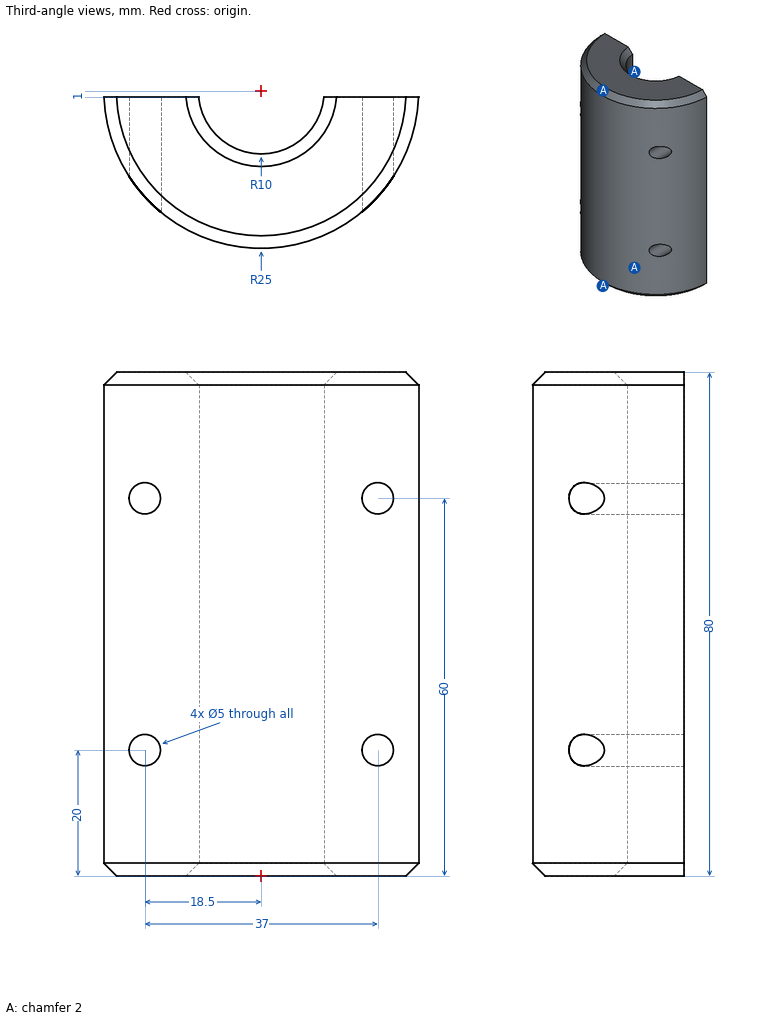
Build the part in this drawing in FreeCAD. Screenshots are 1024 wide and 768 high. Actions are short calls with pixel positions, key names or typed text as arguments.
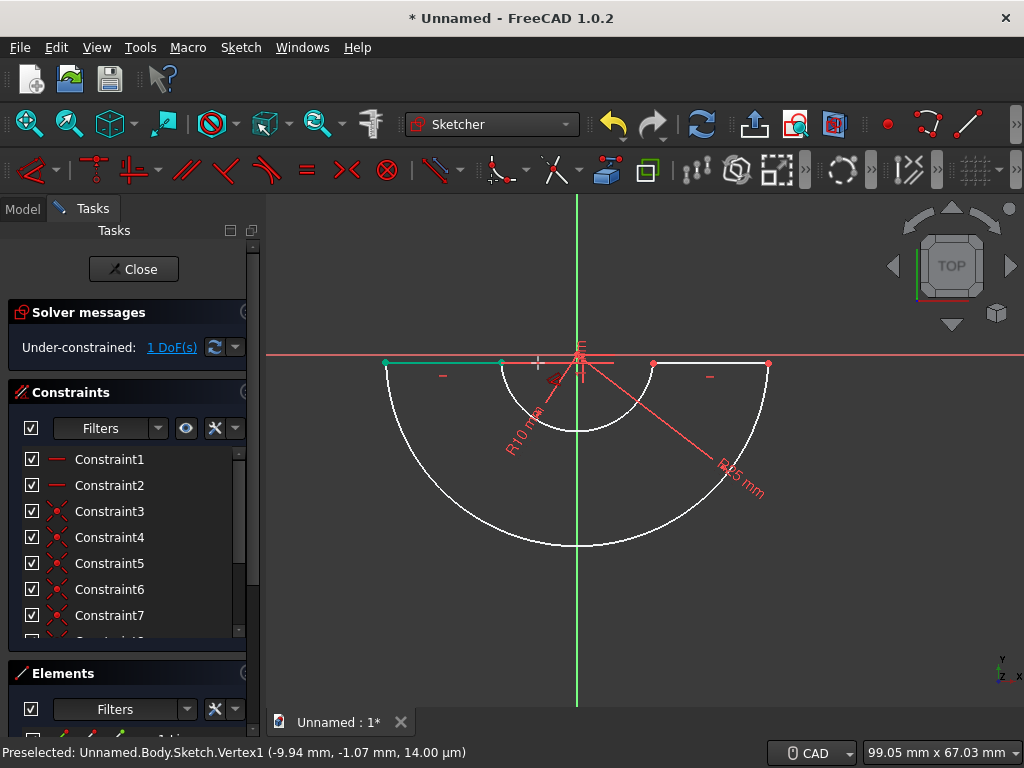
scroll(768, 363, up, 9)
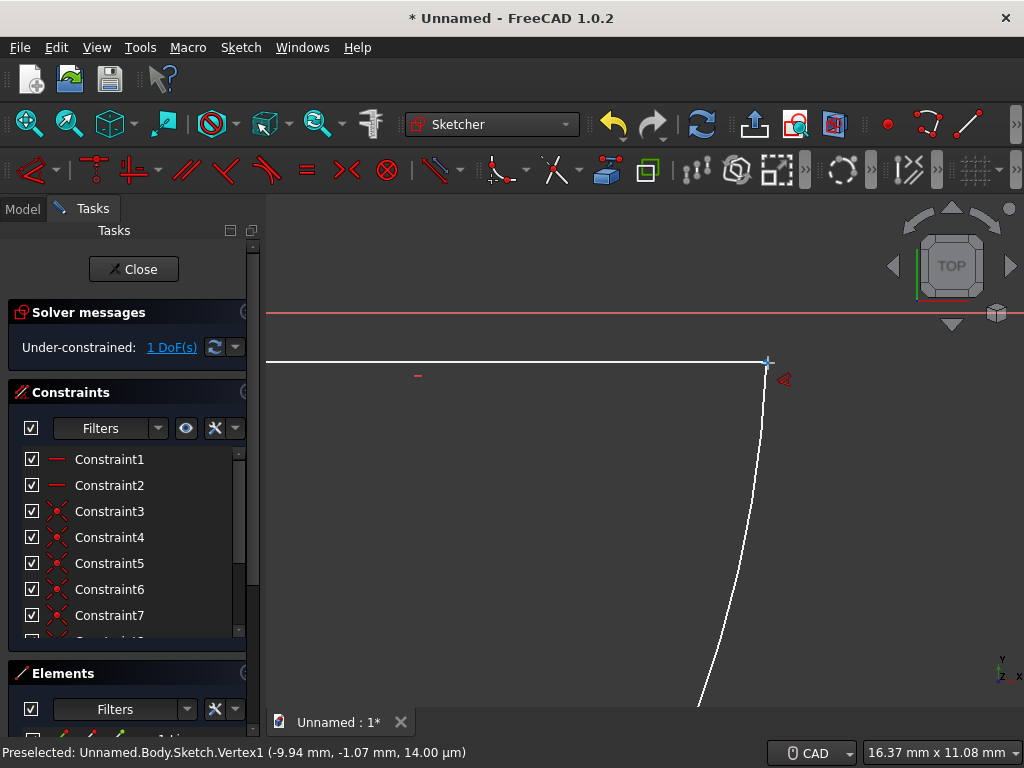
click(766, 362)
click(800, 338)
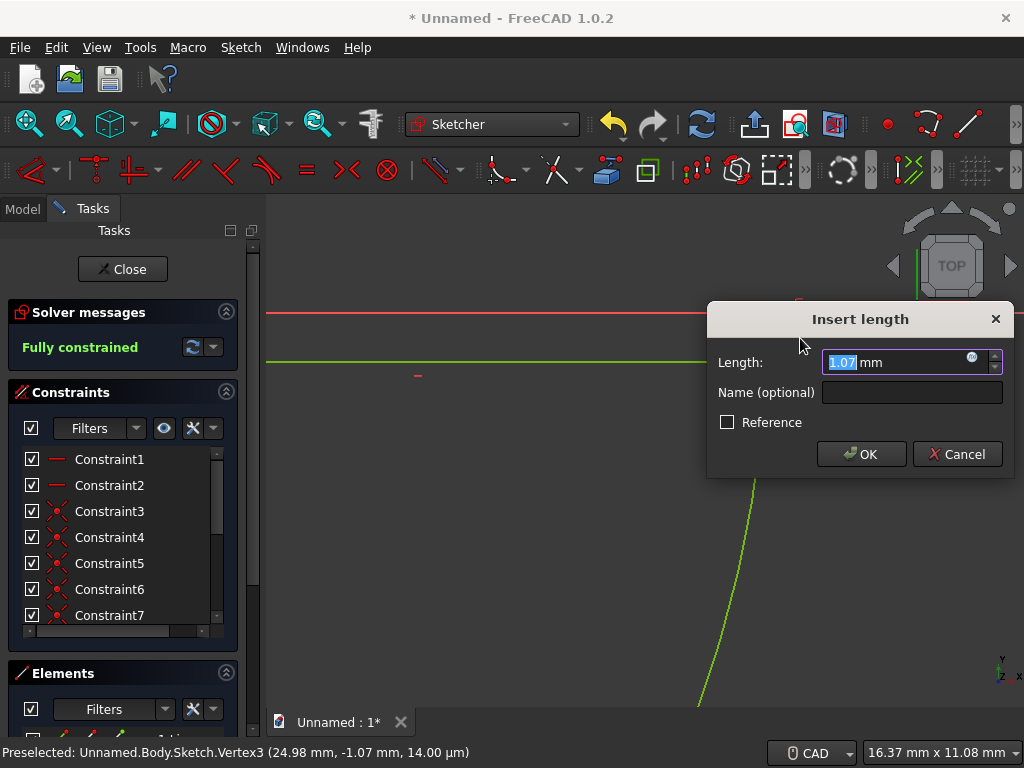
text(1)
key(Return)
key(Escape)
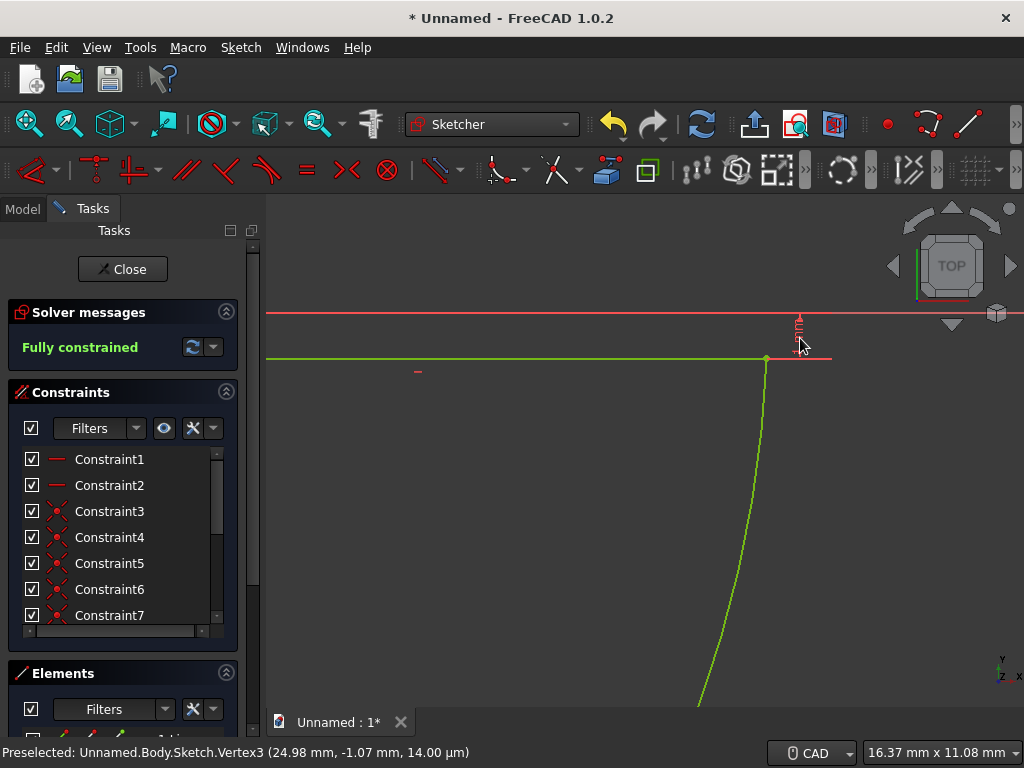
click(123, 269)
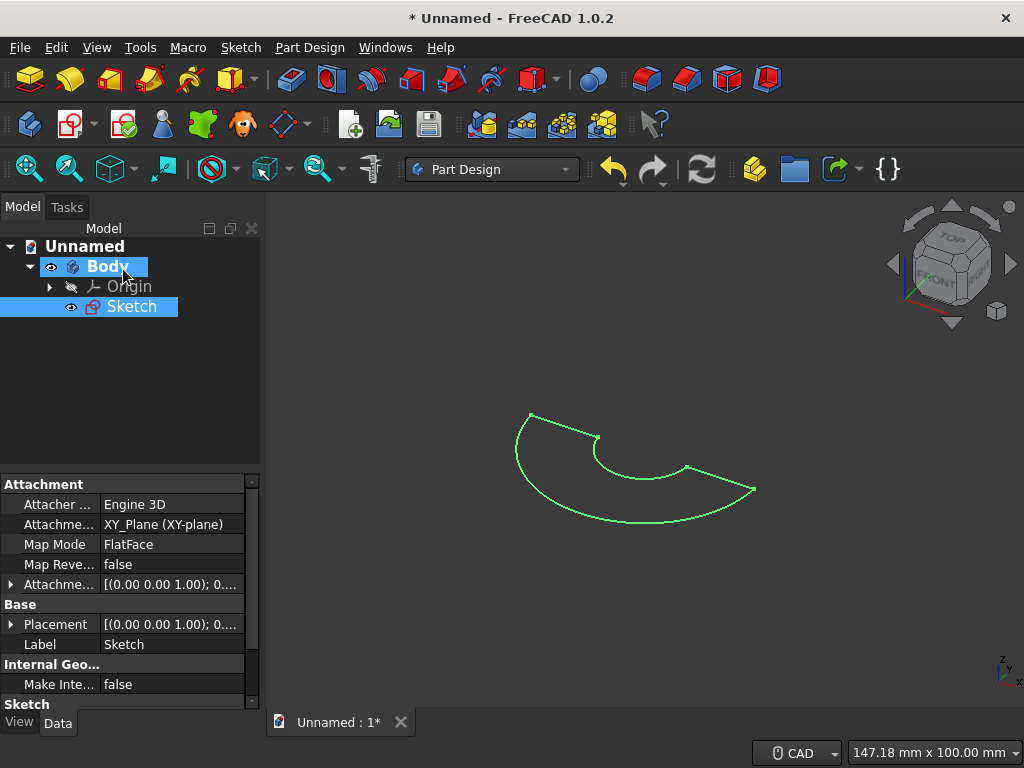
click(30, 80)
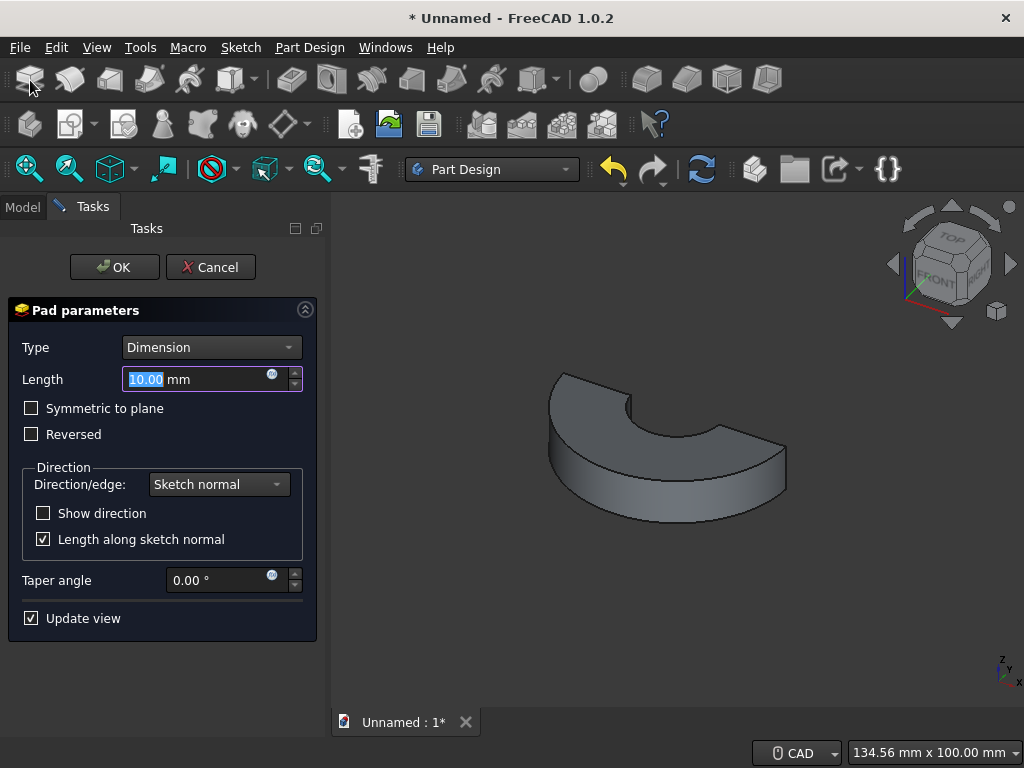
text(80)
key(Tab)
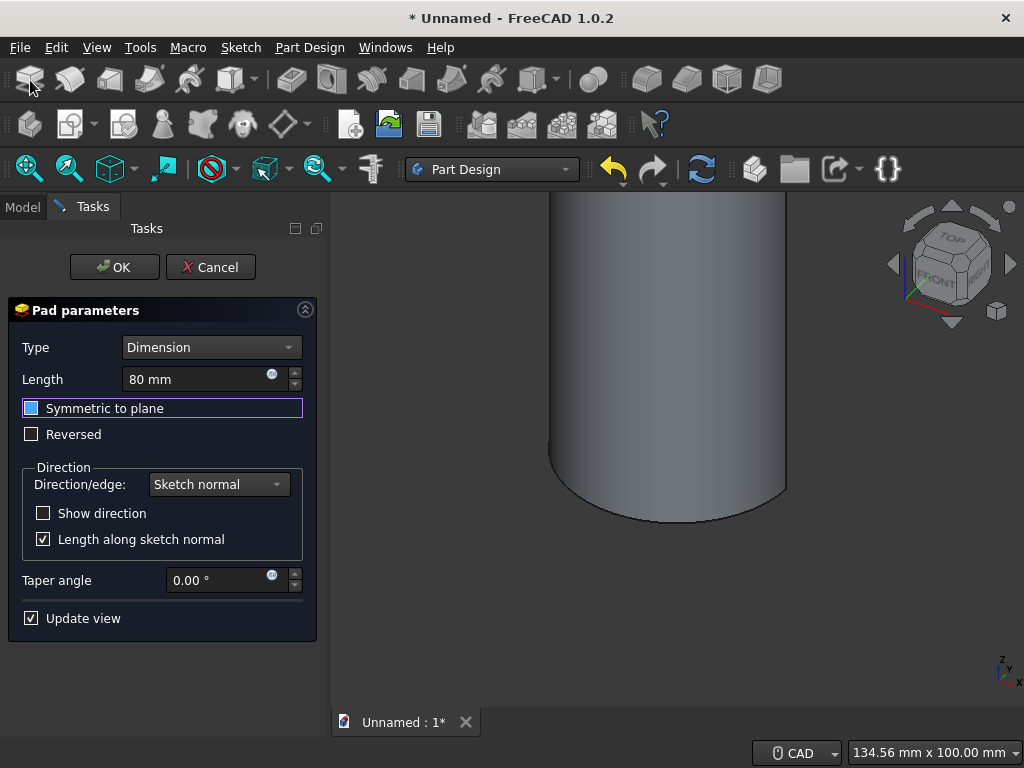
click(115, 267)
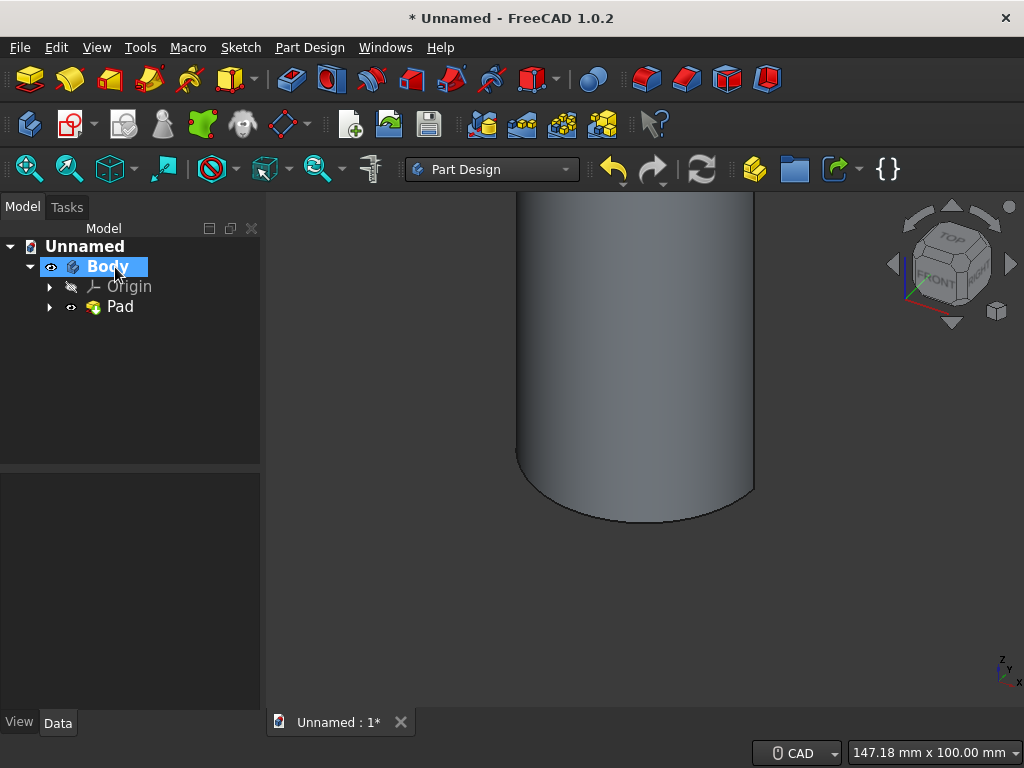
click(30, 170)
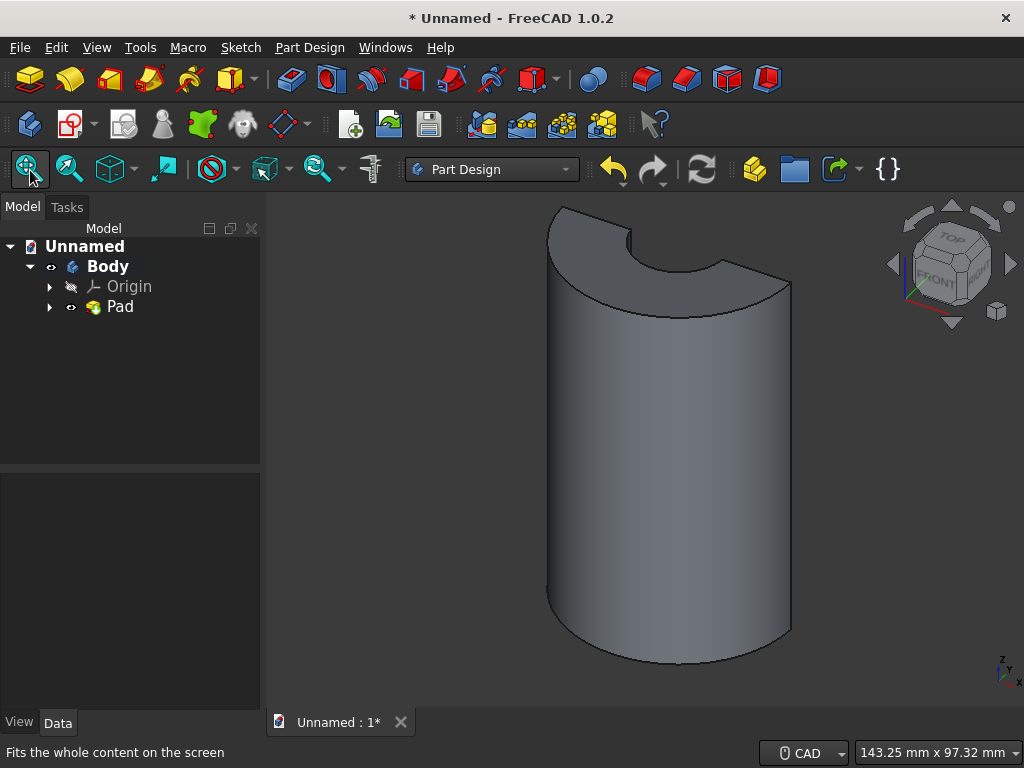
key(4)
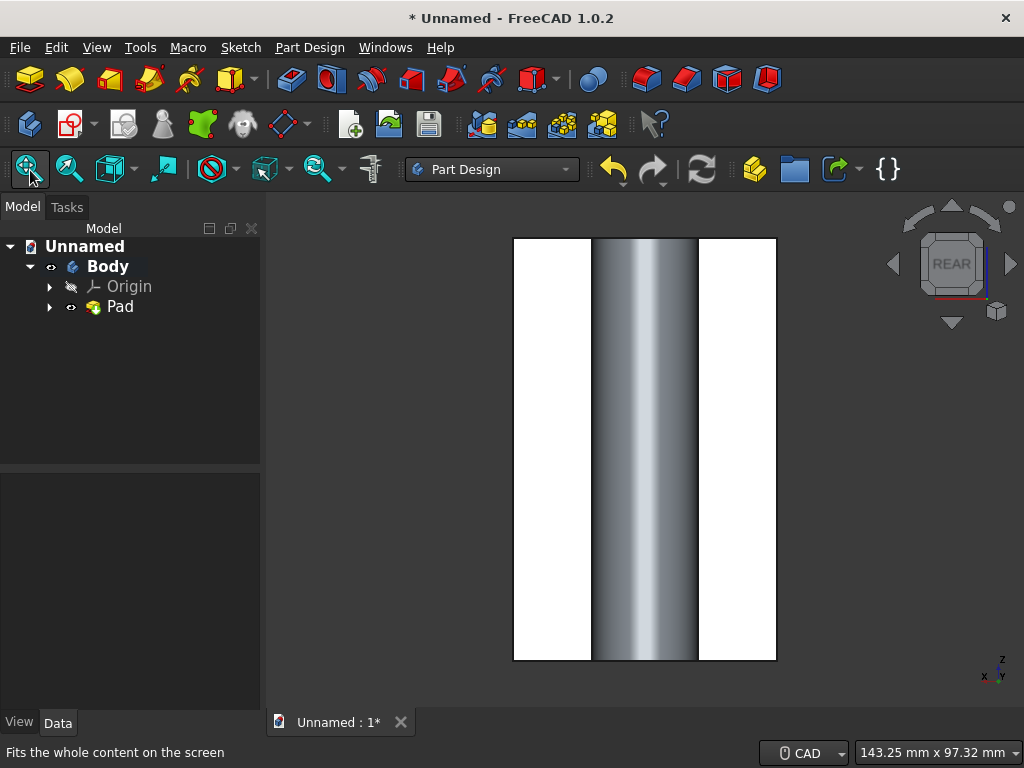
click(737, 328)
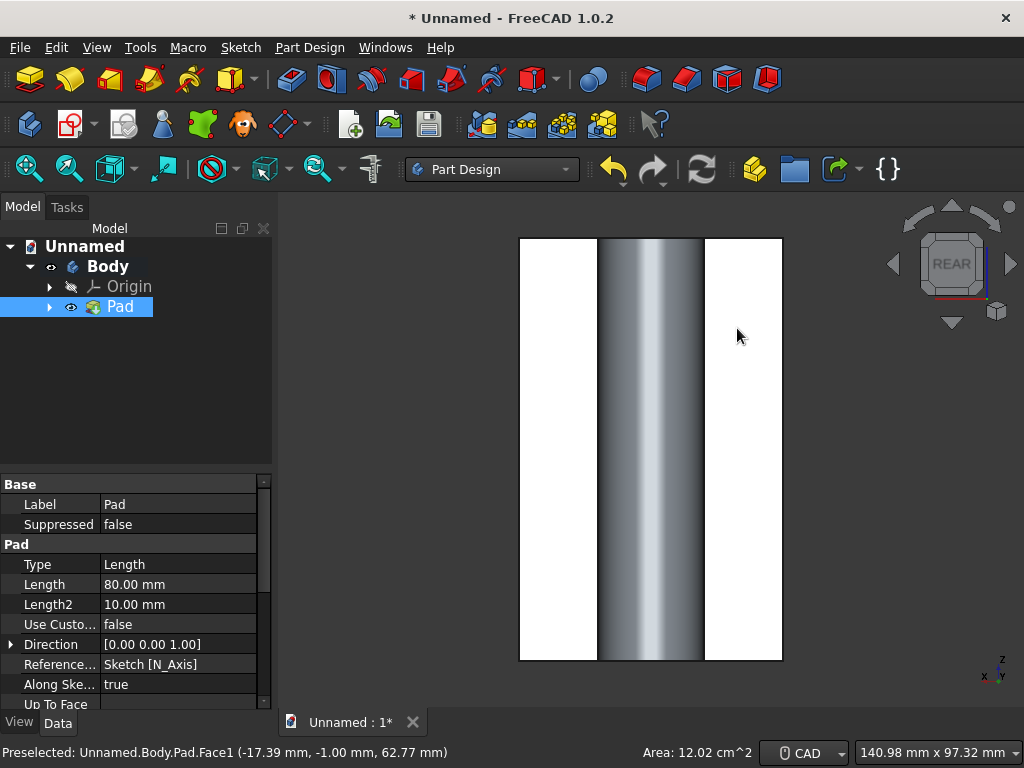
click(70, 124)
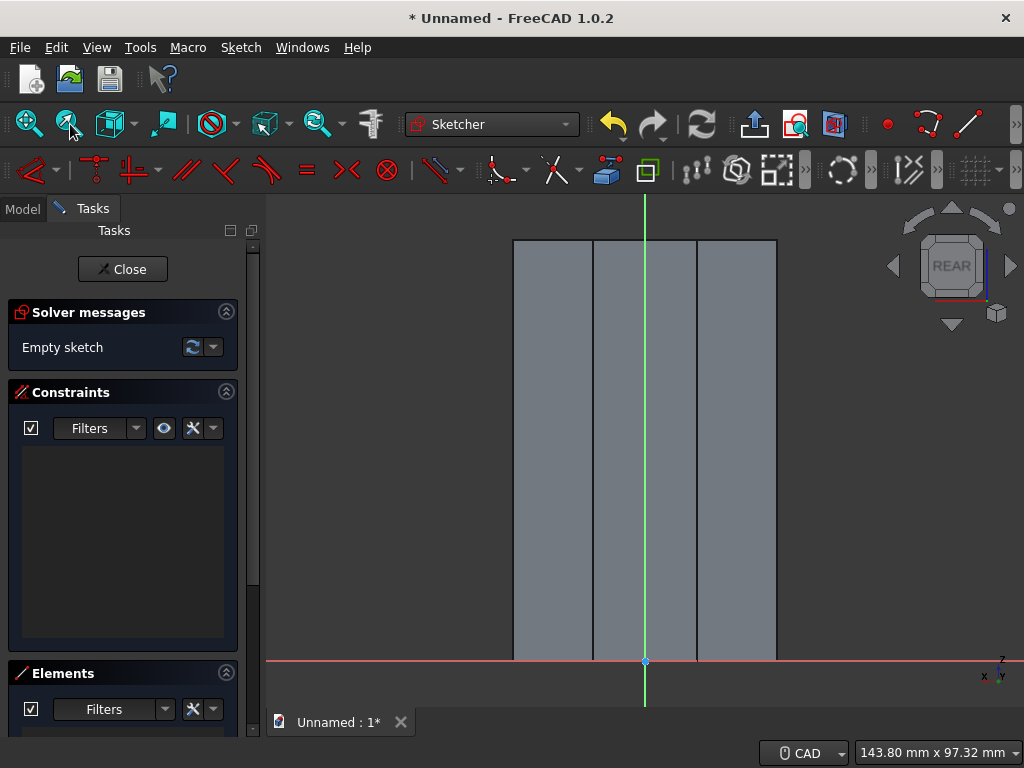
scroll(294, 242, down, 1)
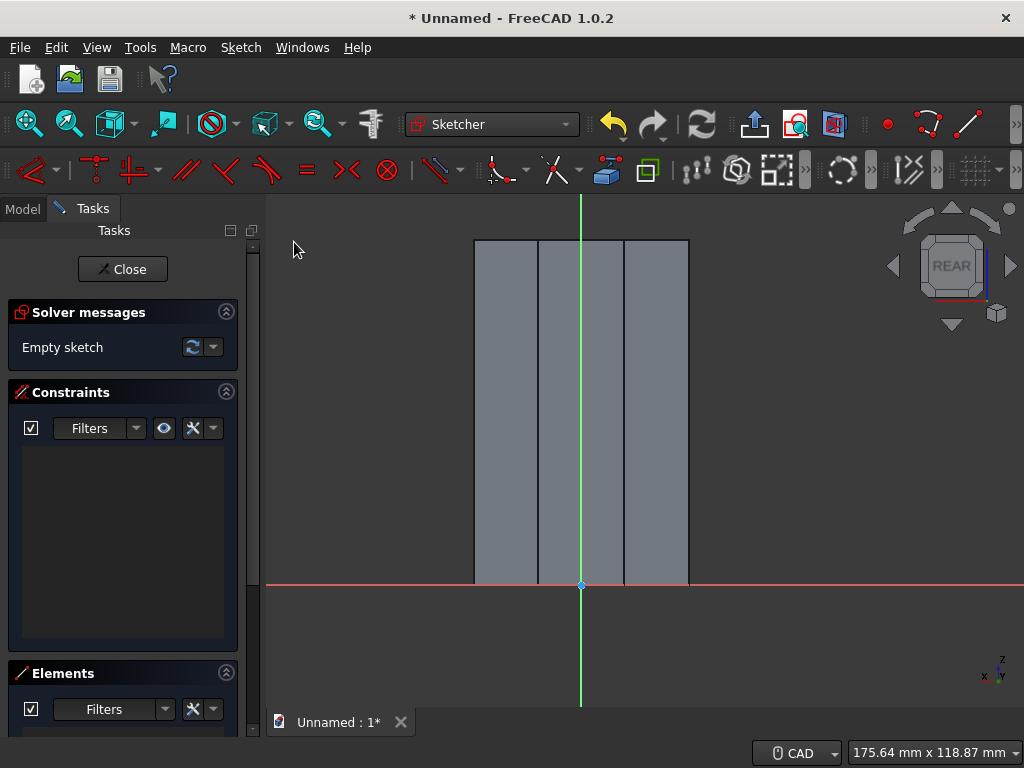
key(g)
key(c)